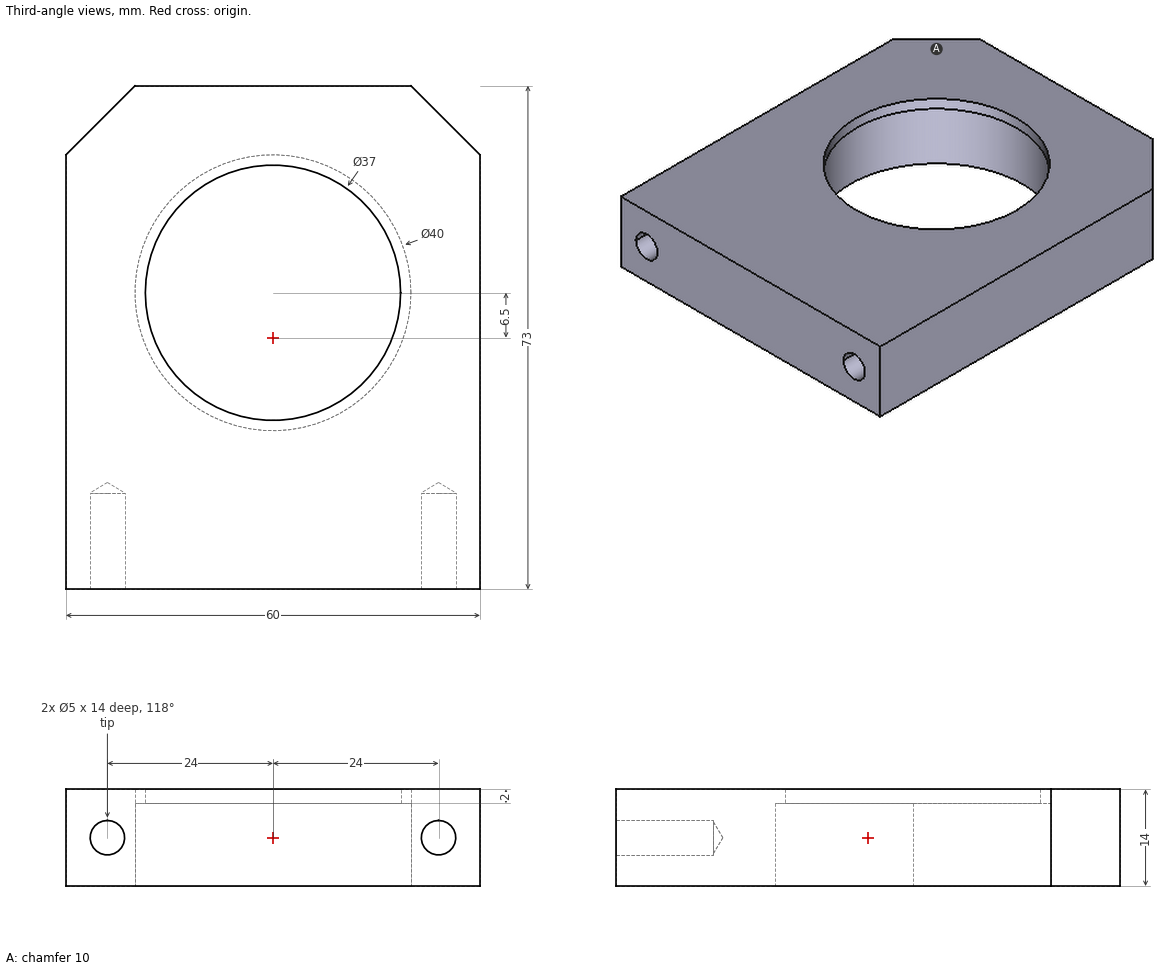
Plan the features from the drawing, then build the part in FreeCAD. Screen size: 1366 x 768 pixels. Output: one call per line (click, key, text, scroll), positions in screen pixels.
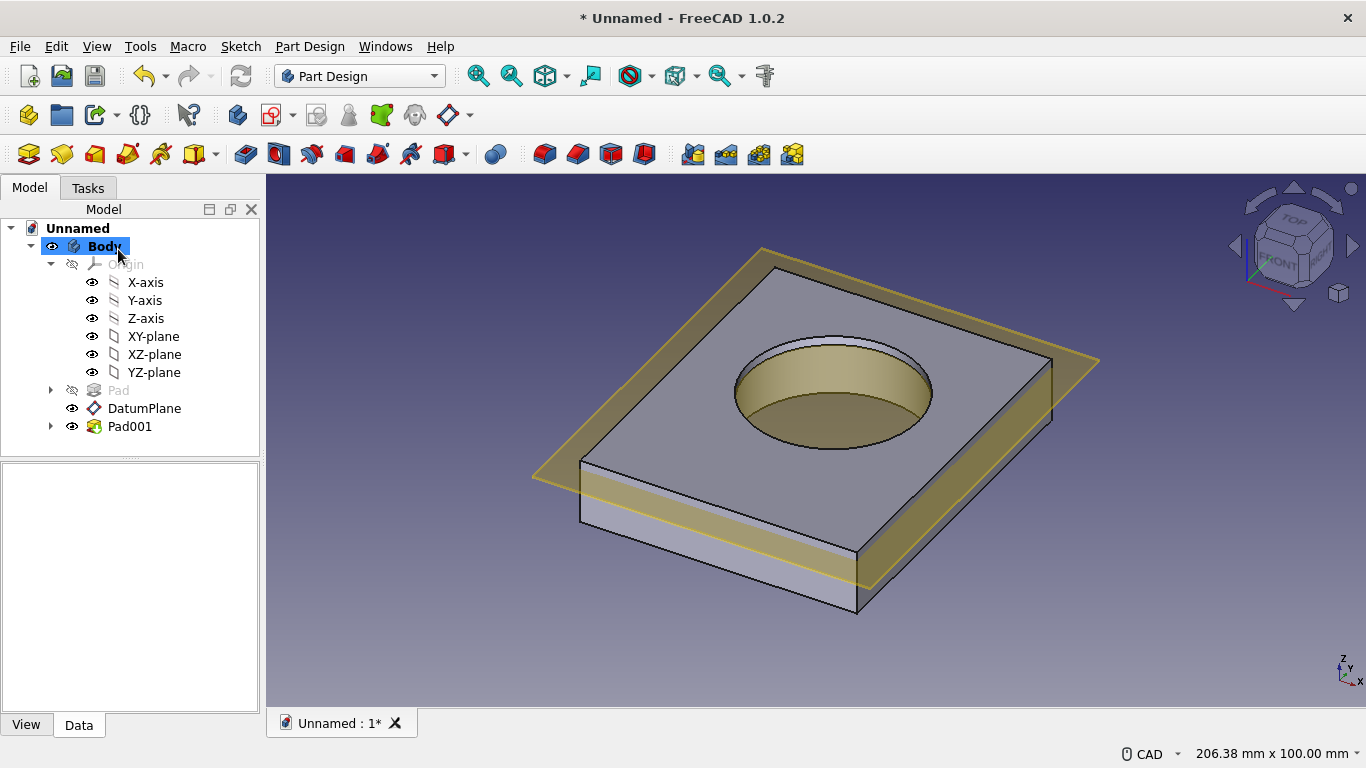
click(117, 408)
key(space)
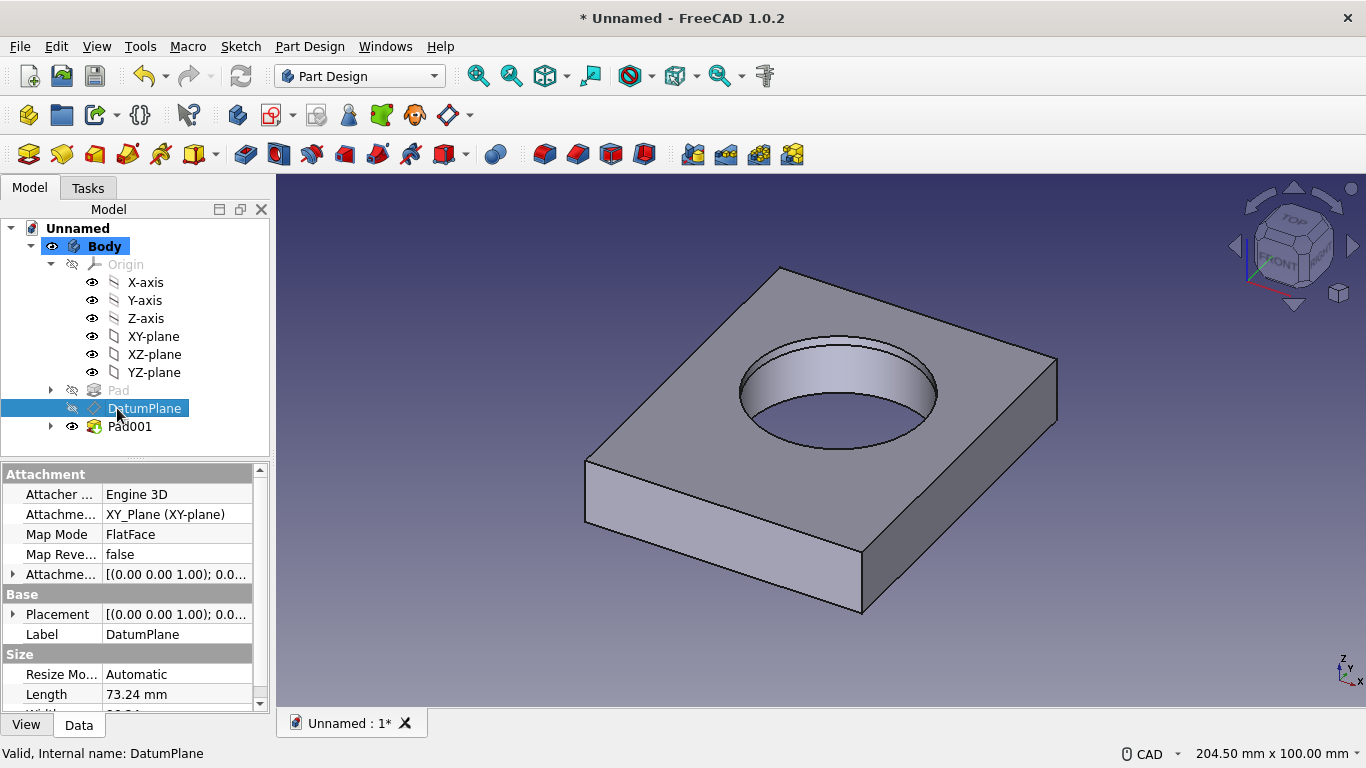
key(0)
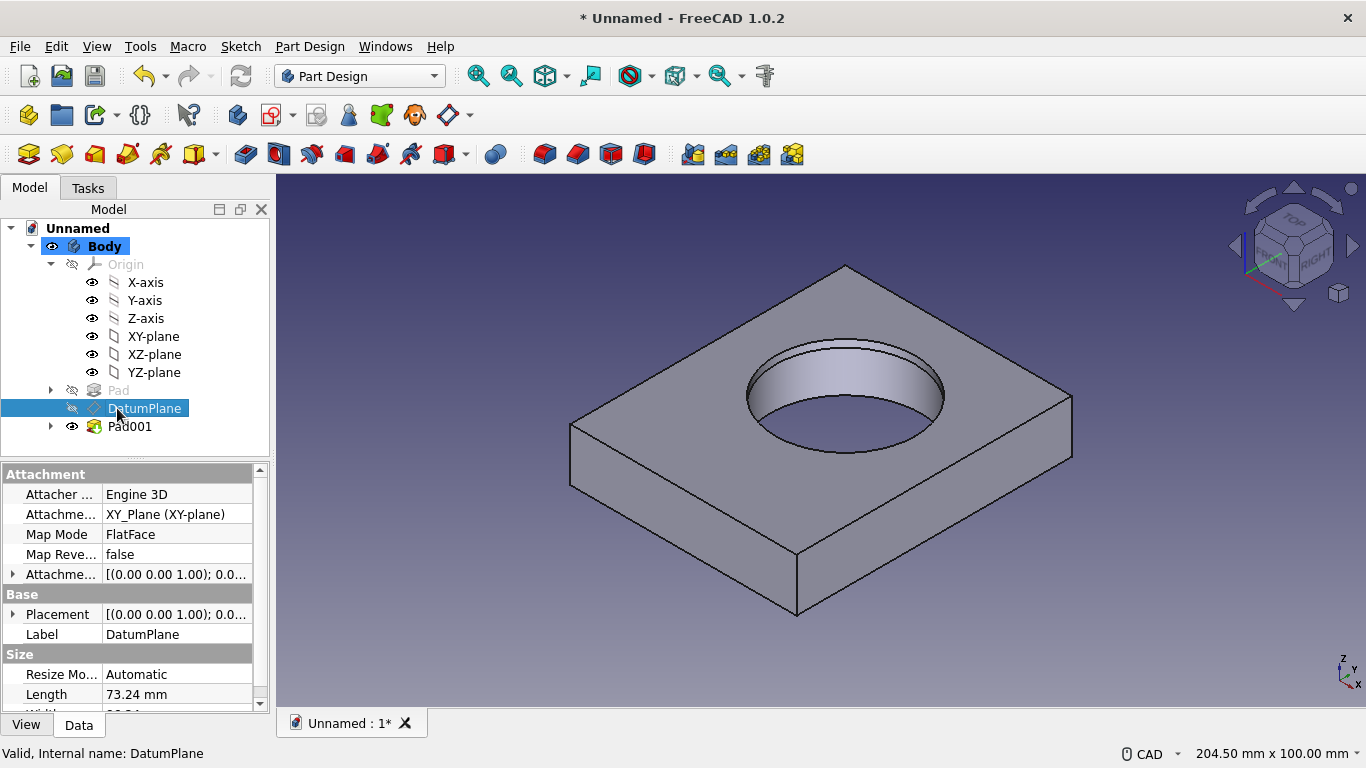
key(2)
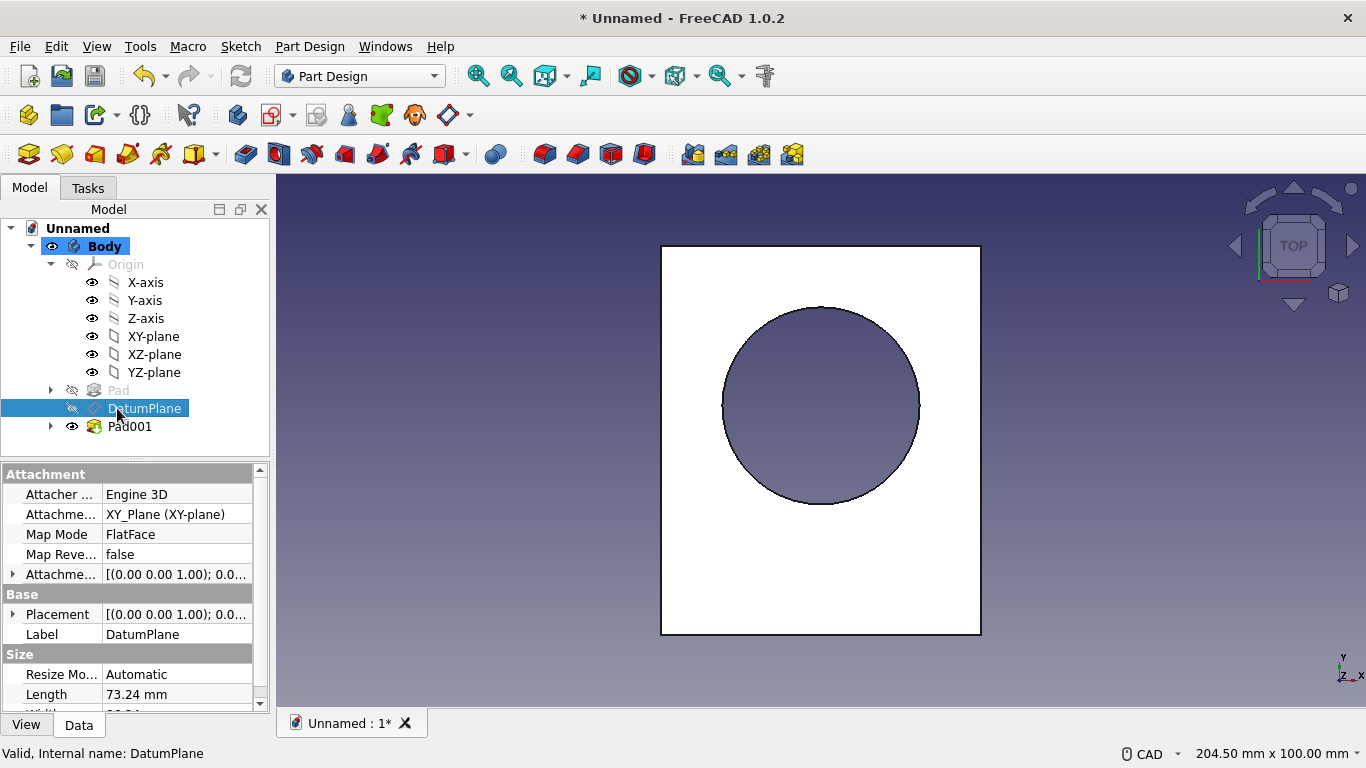
key(1)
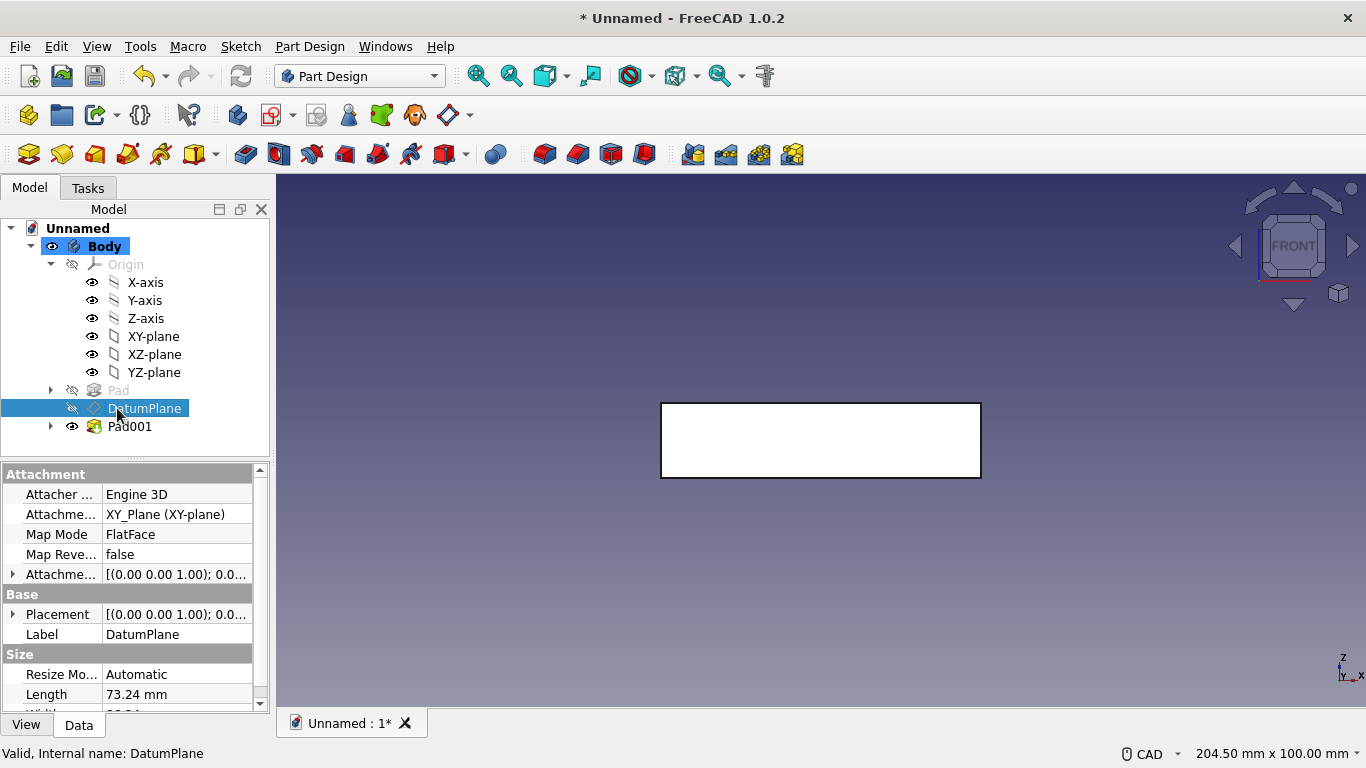
click(479, 76)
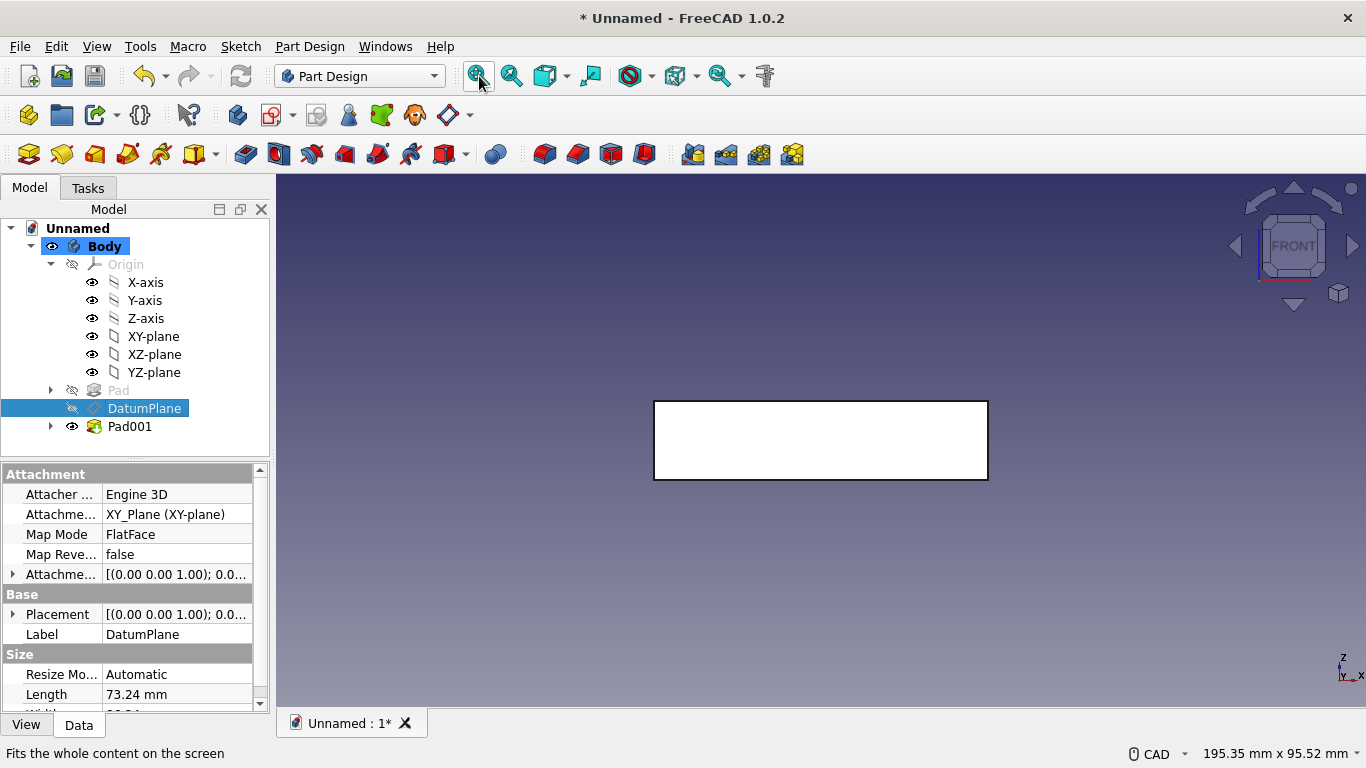
key(3)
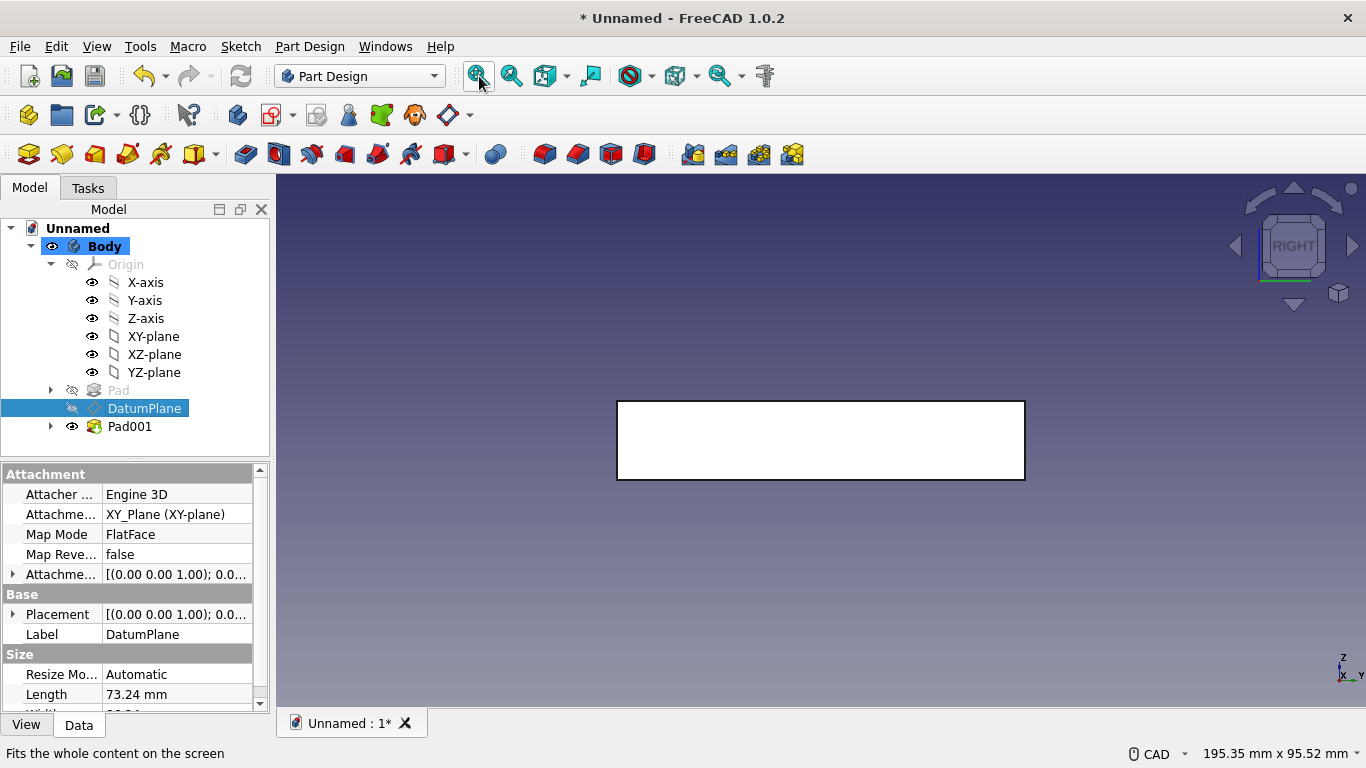
click(479, 76)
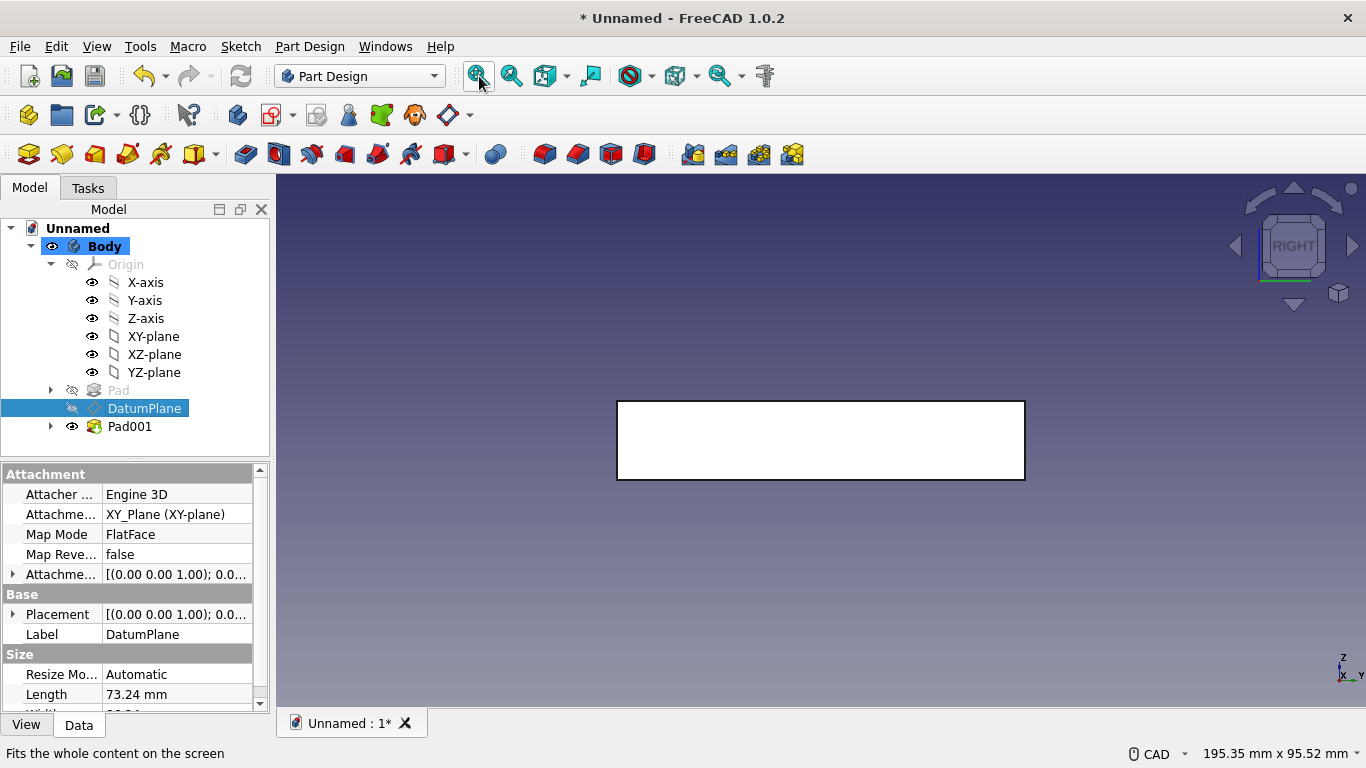
click(1025, 439)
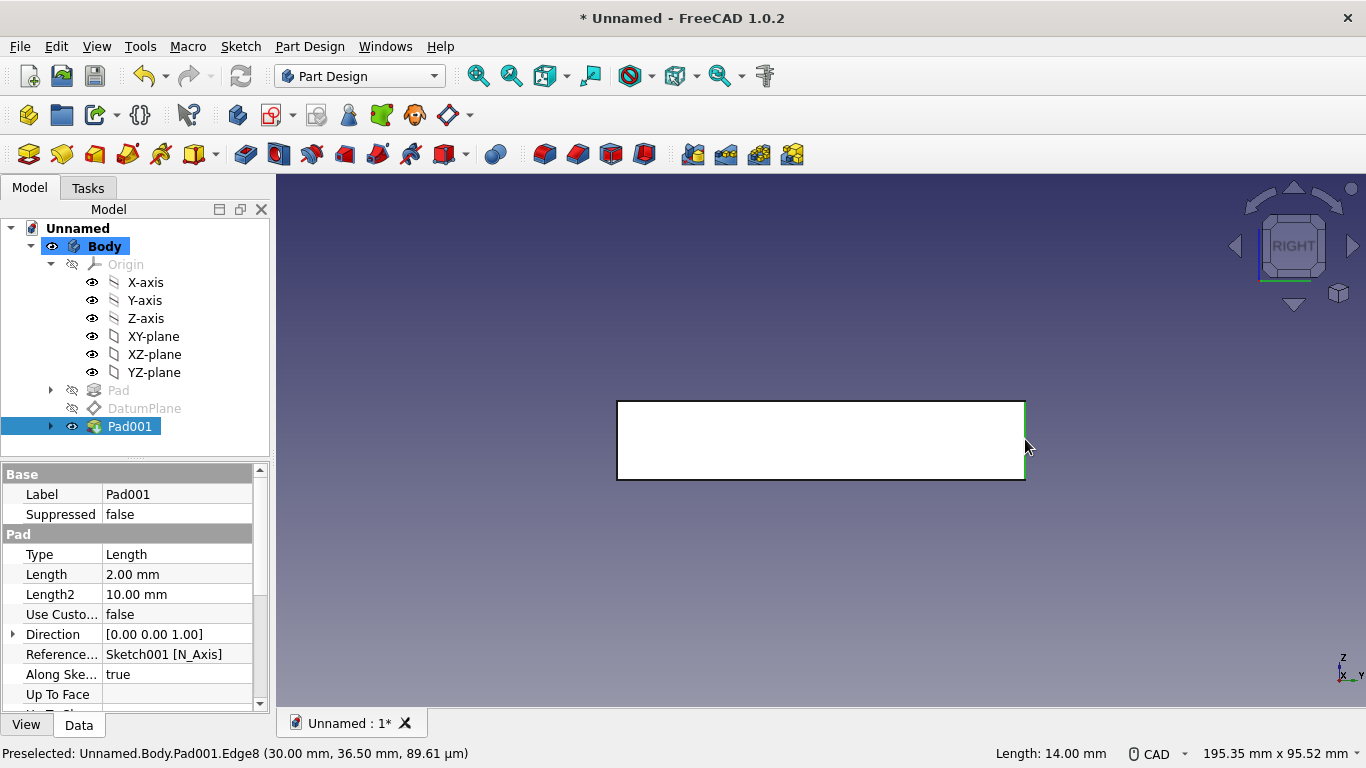
key(5)